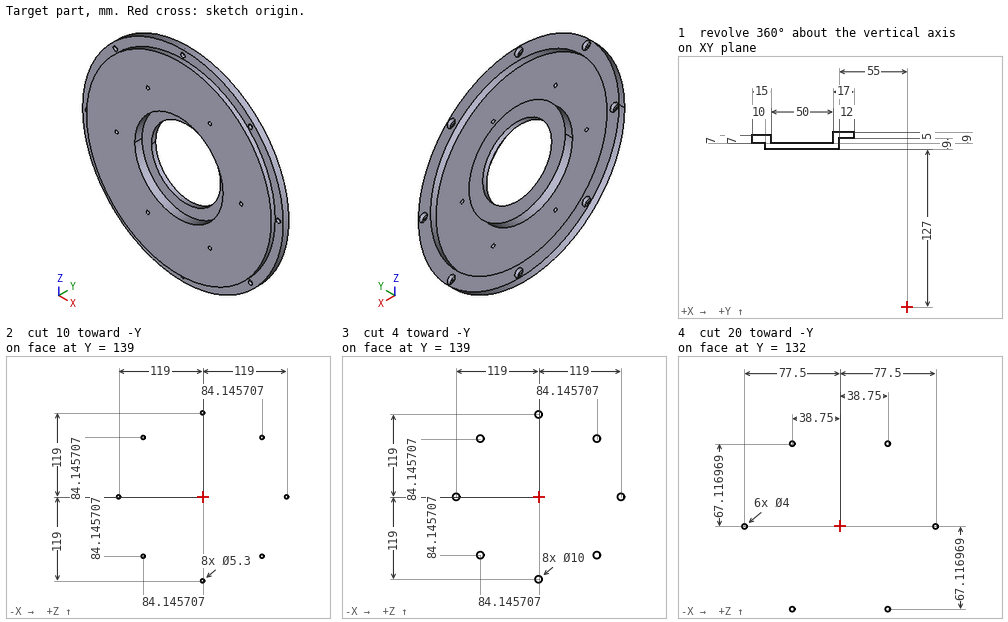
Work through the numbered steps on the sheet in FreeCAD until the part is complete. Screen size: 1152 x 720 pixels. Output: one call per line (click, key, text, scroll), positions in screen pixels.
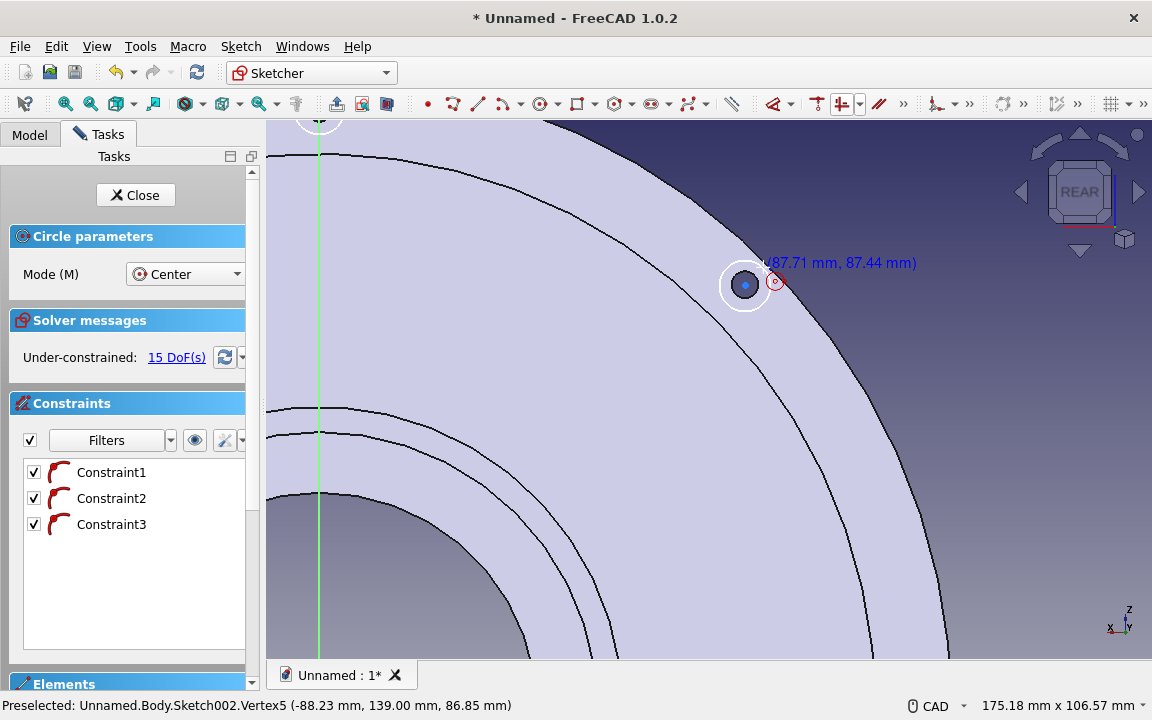
scroll(746, 285, down, 7)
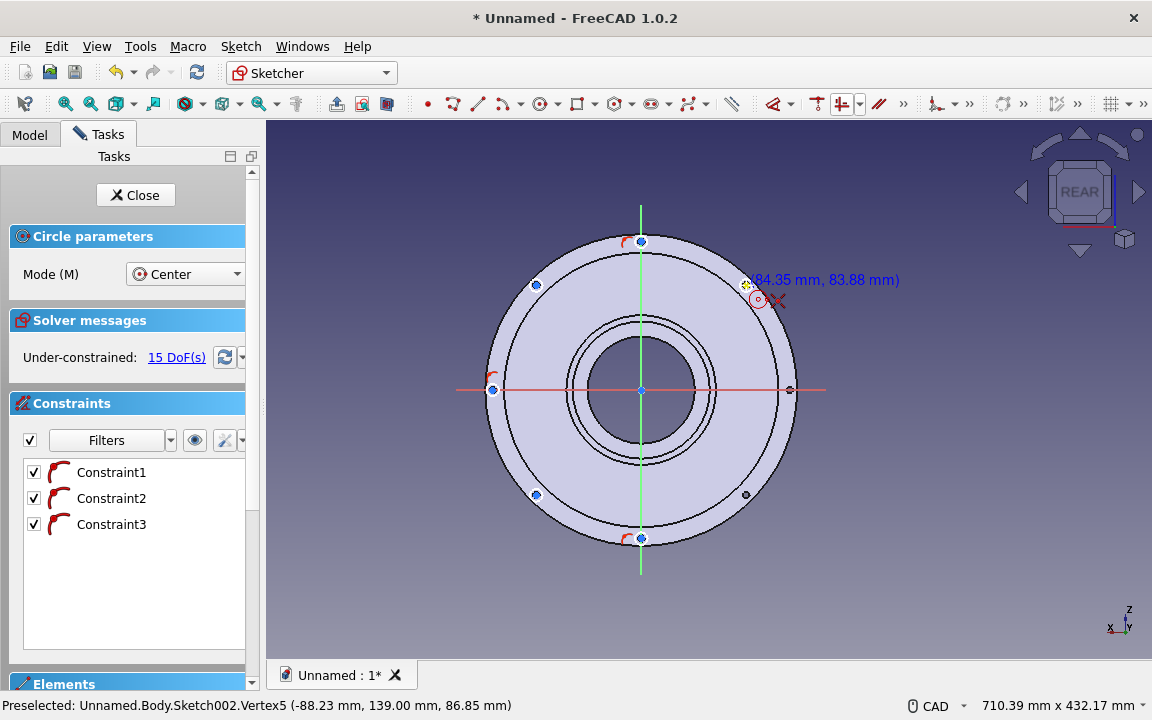
scroll(790, 390, up, 7)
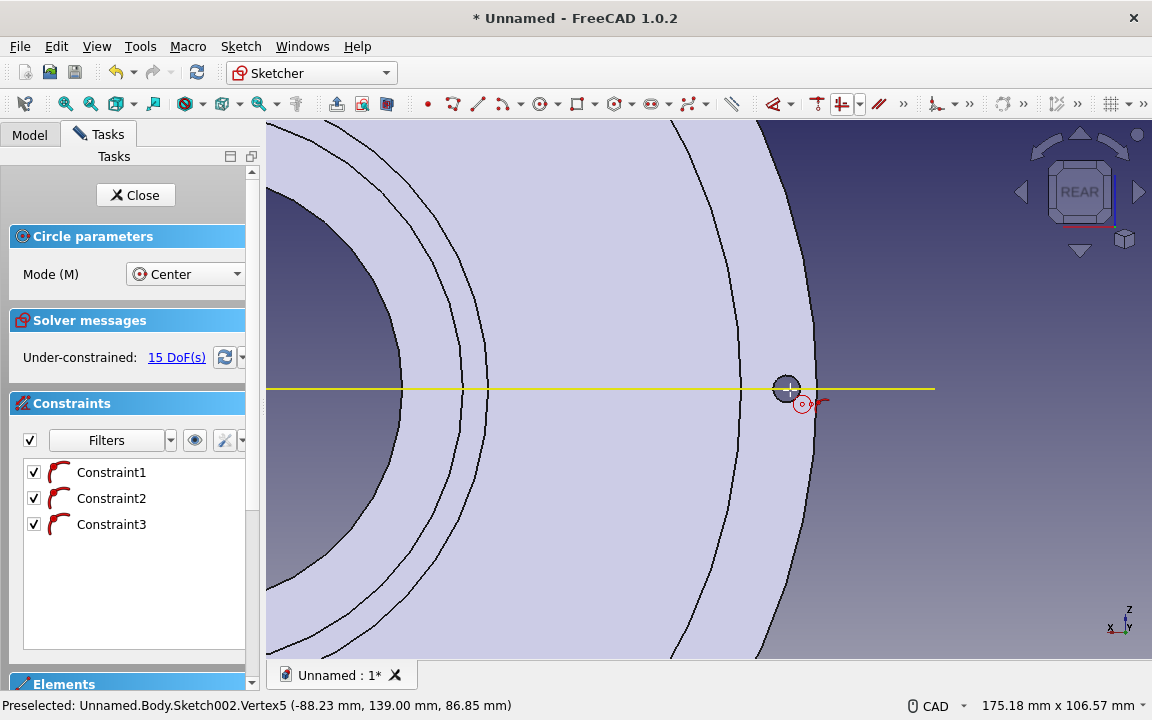
click(787, 389)
click(805, 371)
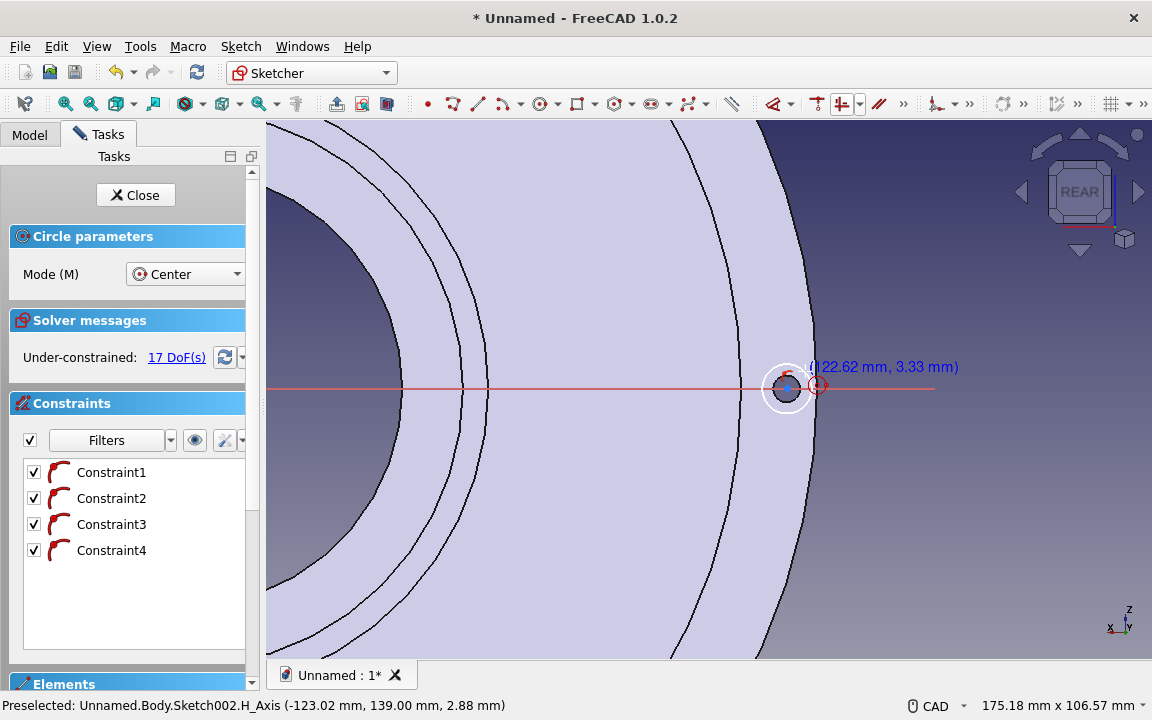
scroll(790, 390, down, 7)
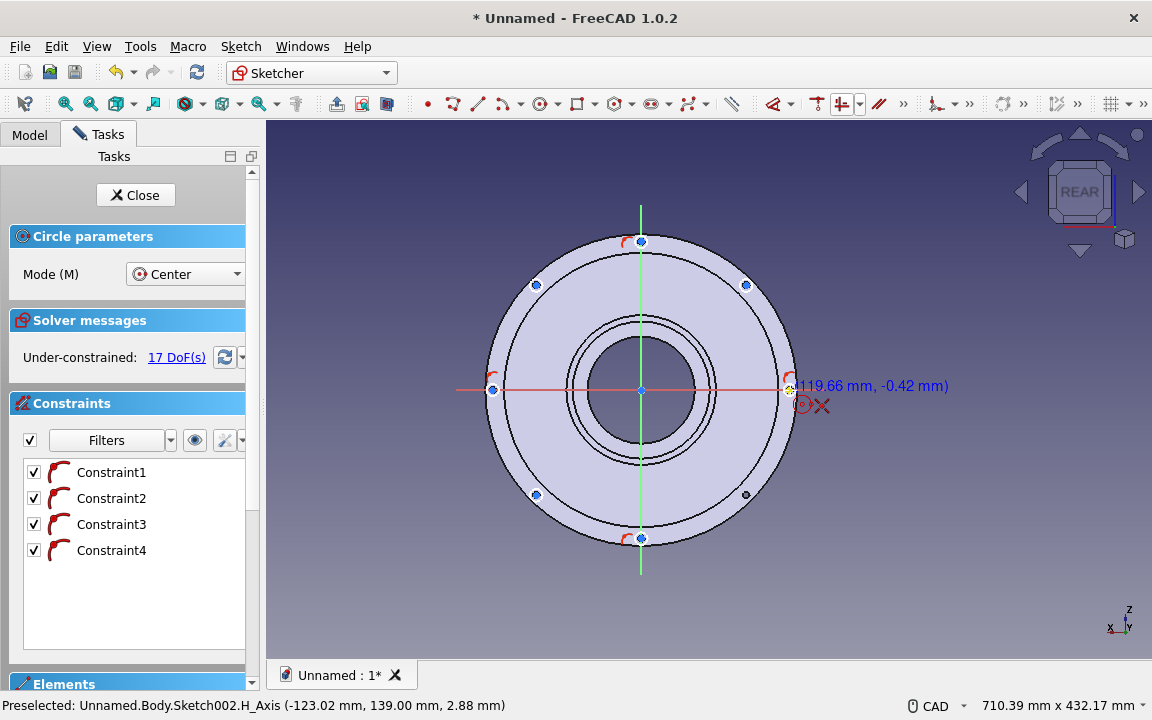
scroll(746, 495, up, 7)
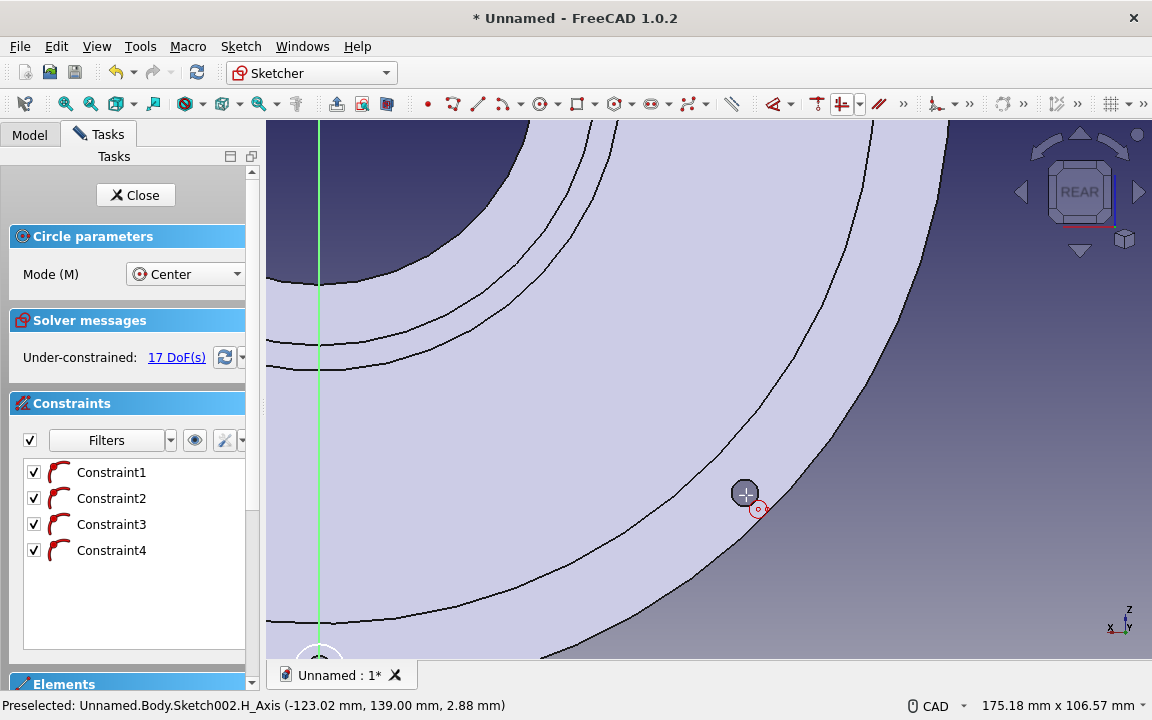
click(745, 493)
click(763, 475)
key(Escape)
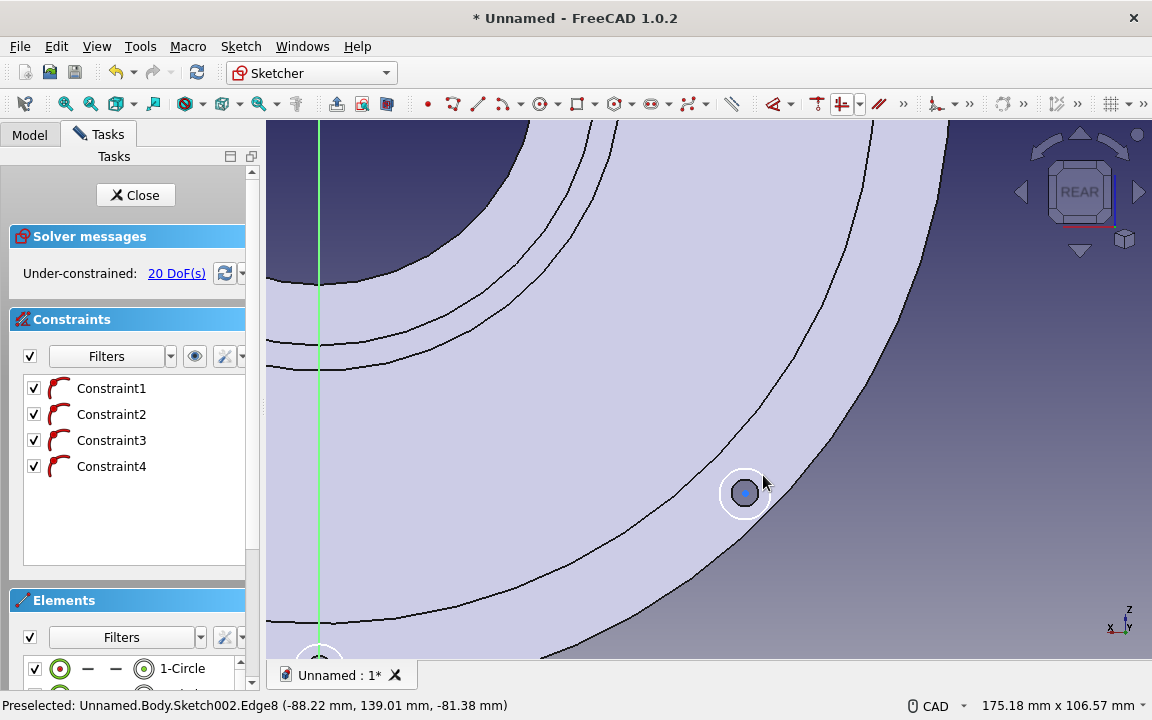
scroll(746, 495, down, 7)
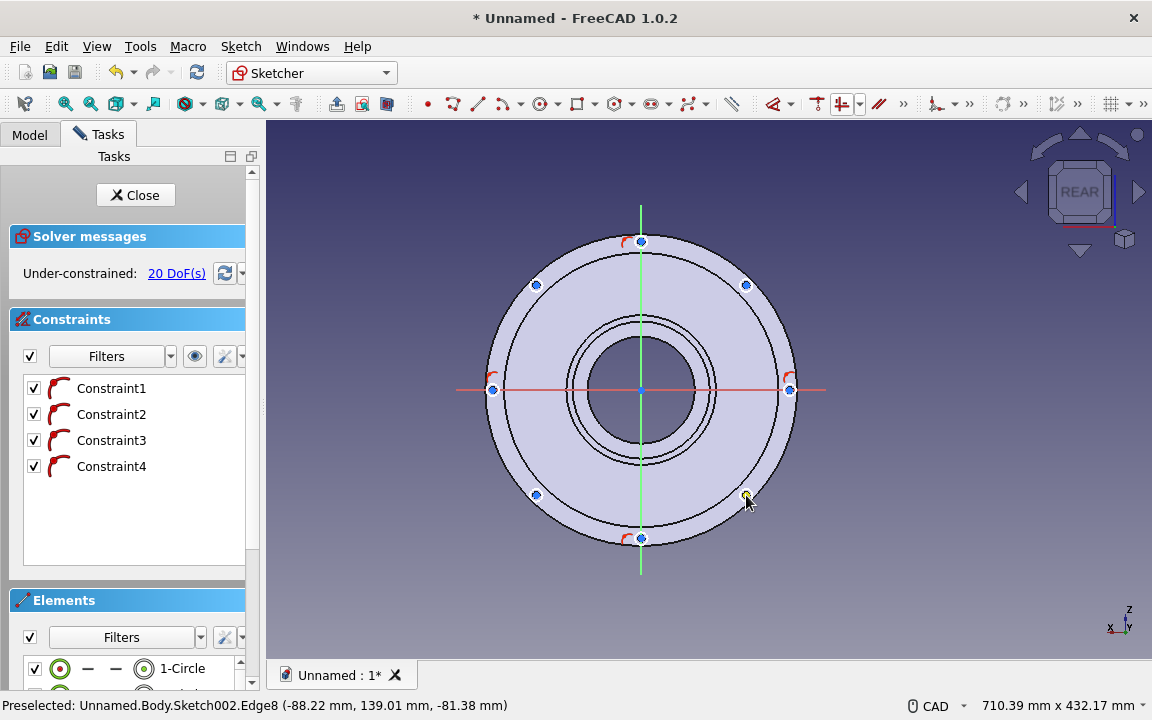
scroll(646, 534, up, 6)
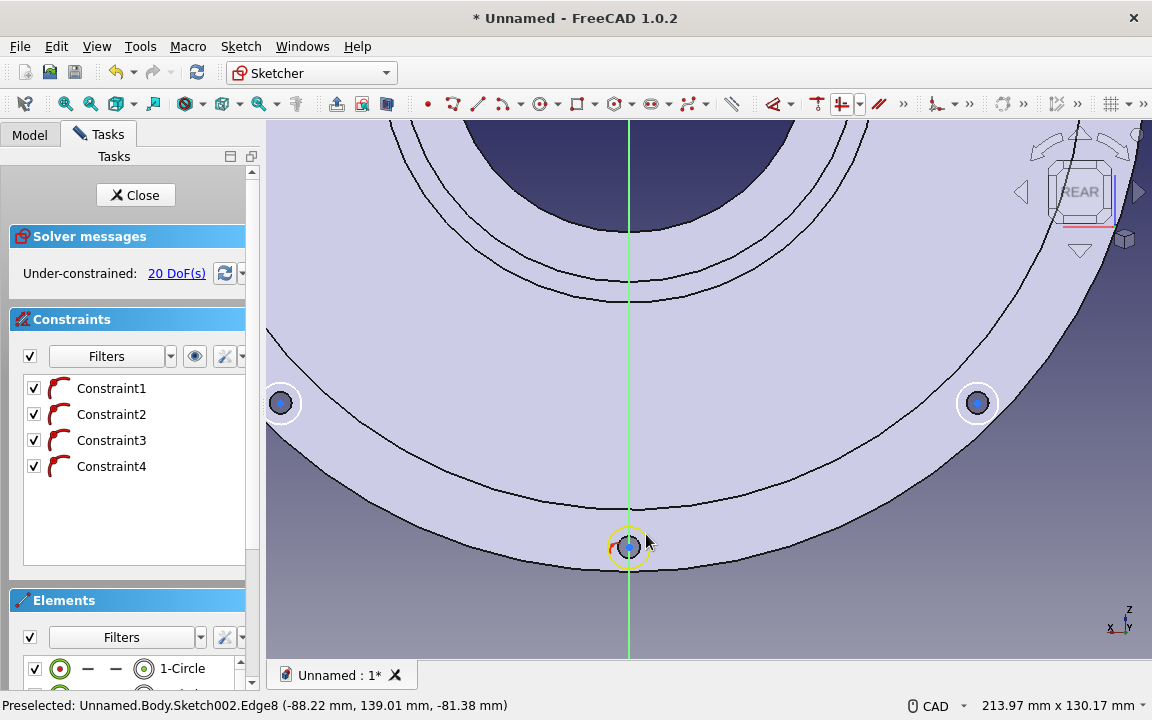
click(644, 533)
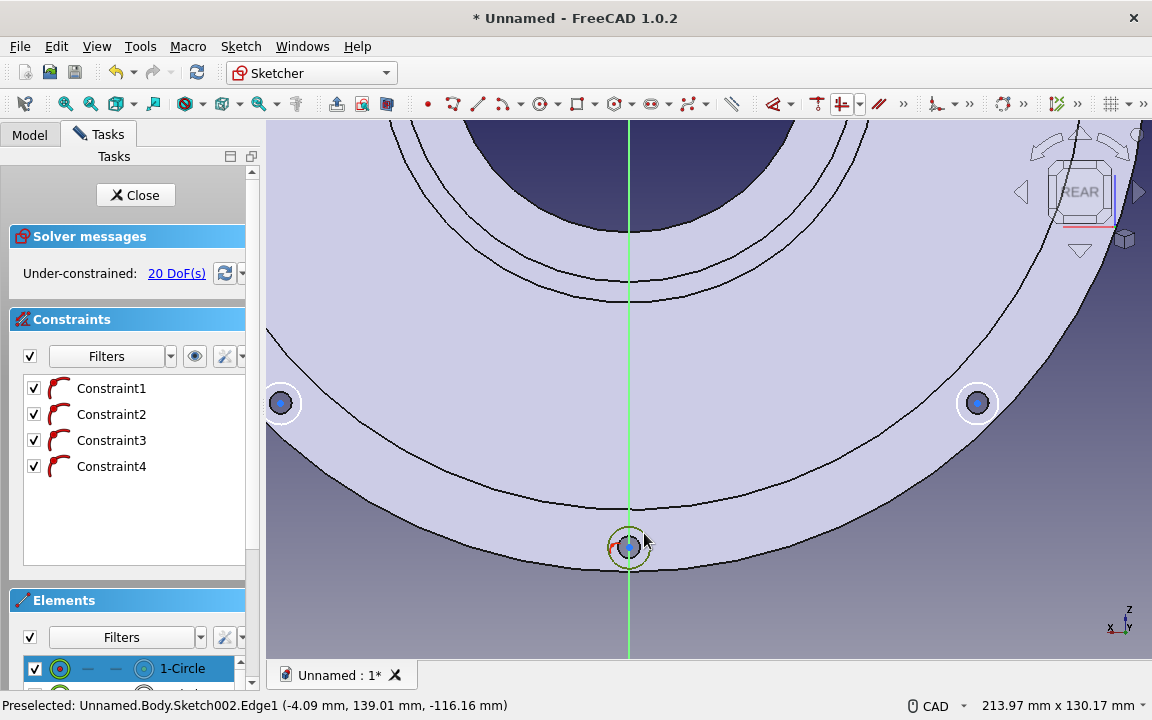
click(295, 389)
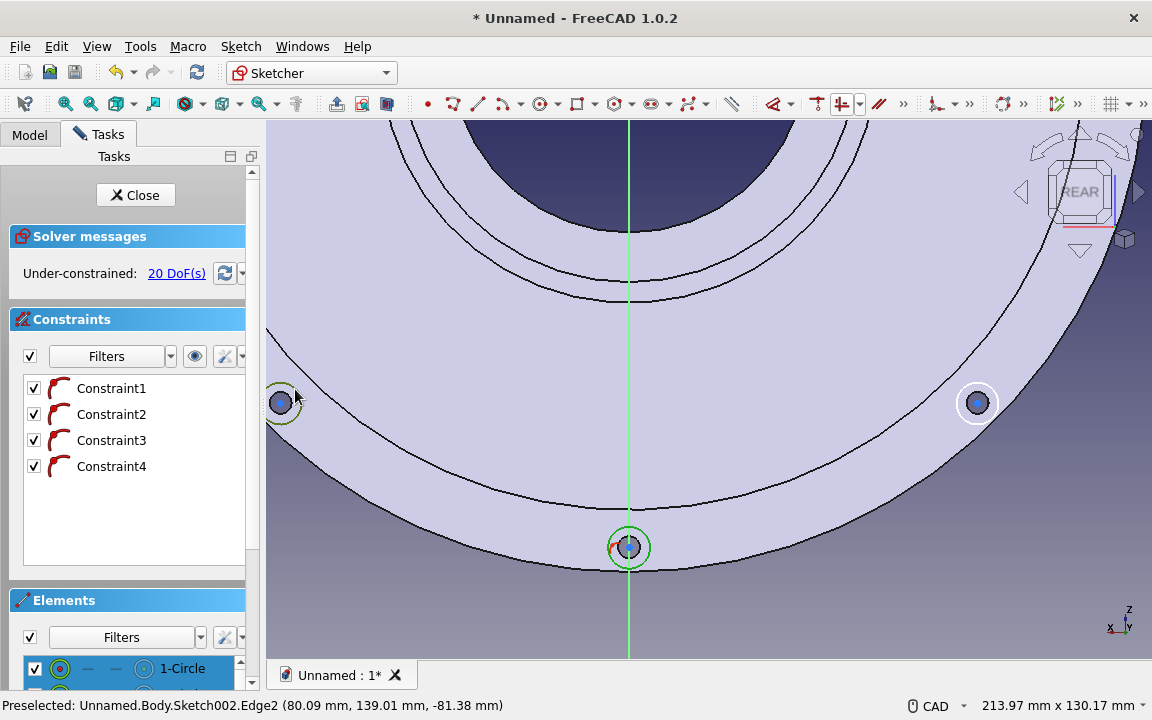
scroll(645, 534, down, 6)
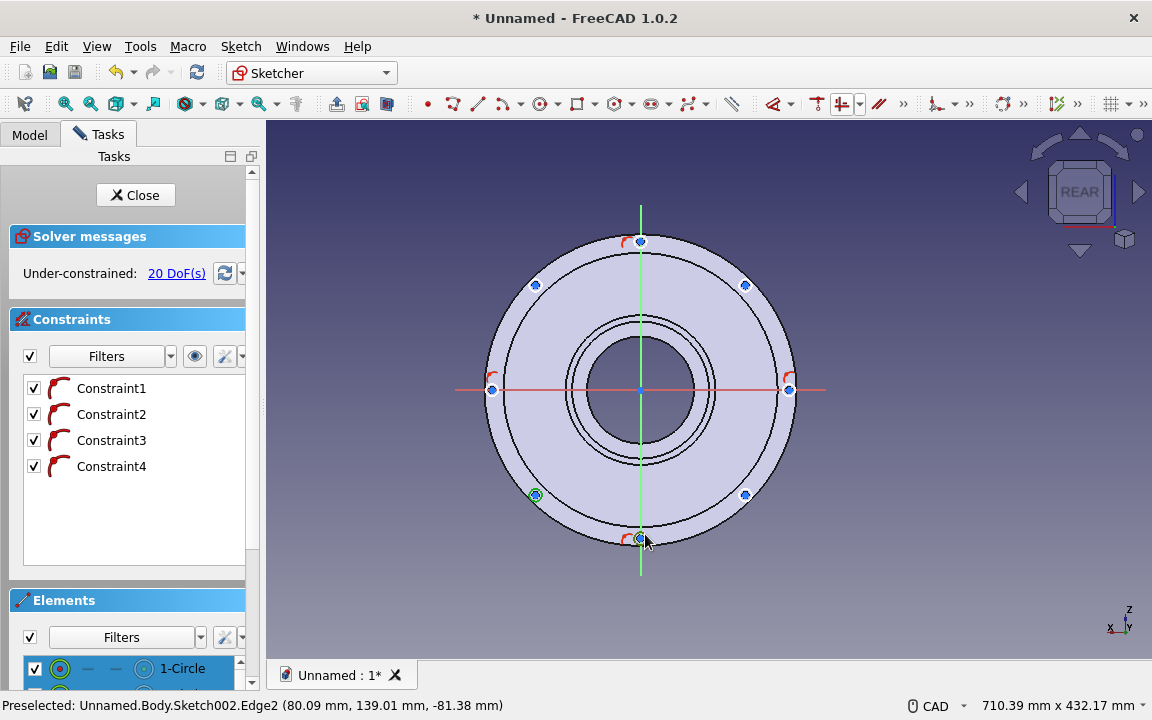
scroll(496, 386, up, 6)